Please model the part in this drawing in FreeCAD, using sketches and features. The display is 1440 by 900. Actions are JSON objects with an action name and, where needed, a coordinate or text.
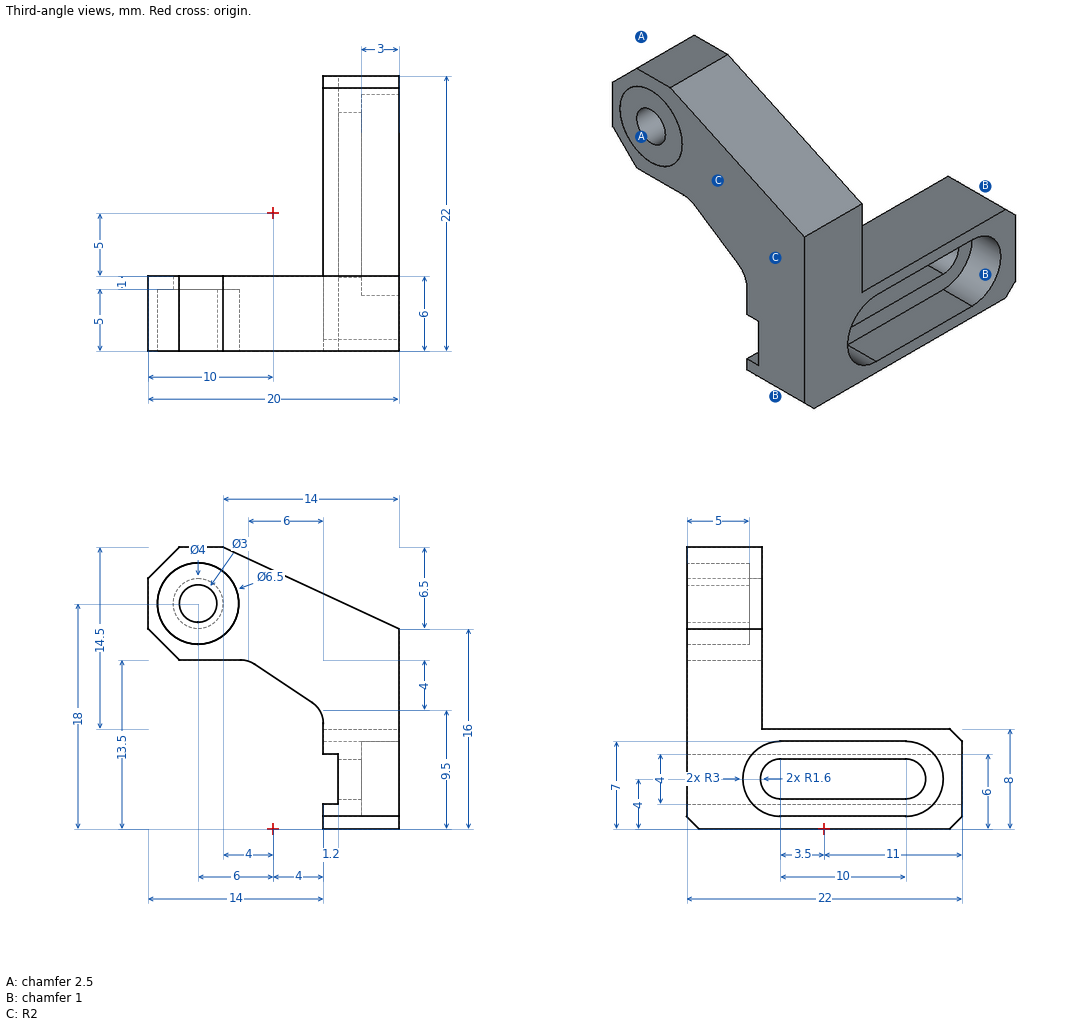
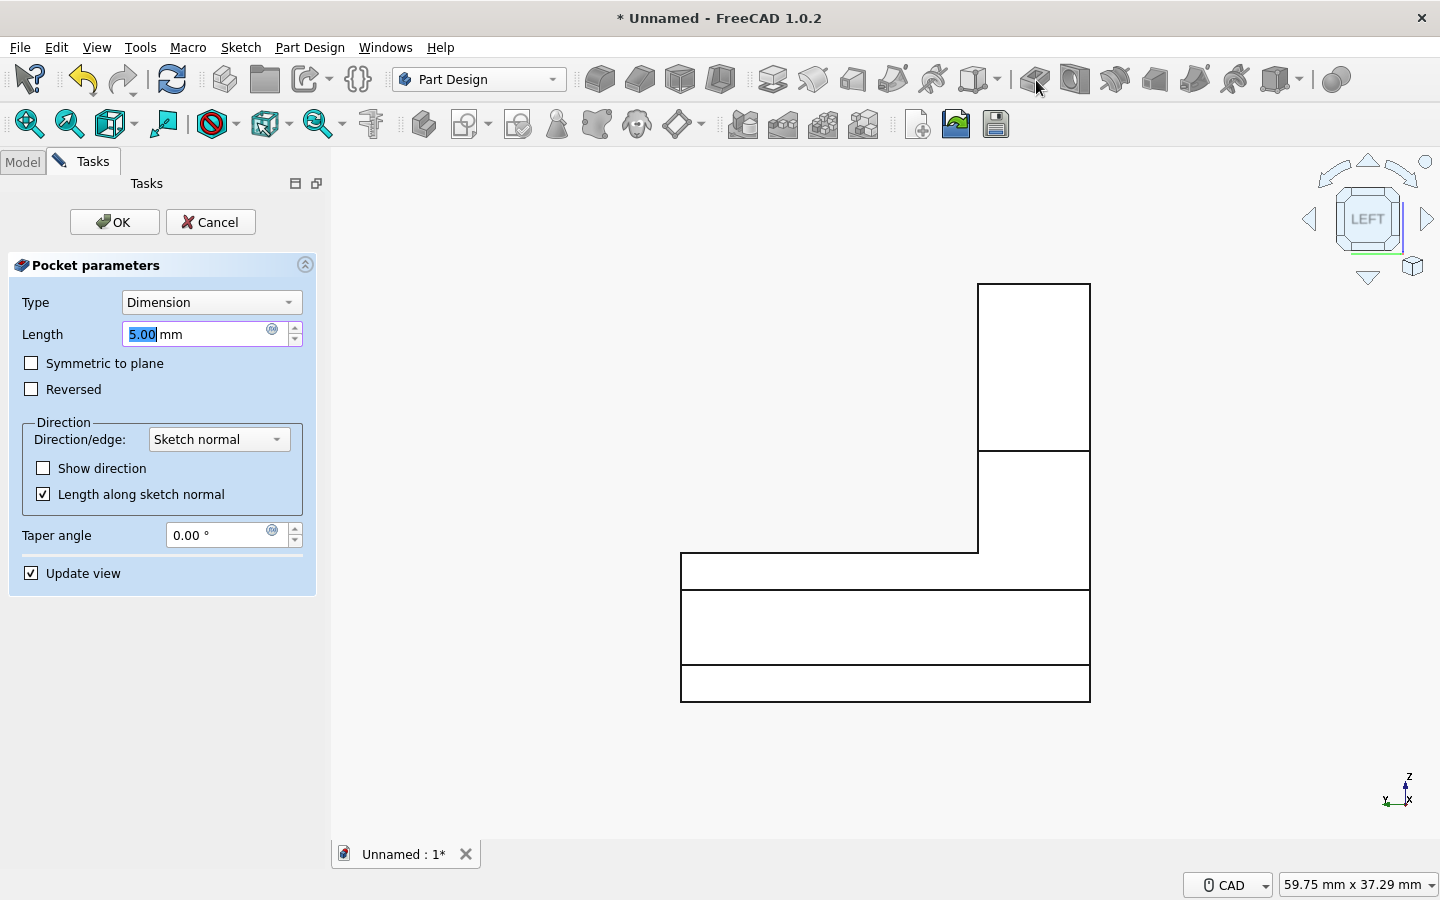
{"action": "type", "text": "1.2"}
{"action": "key", "text": "Tab"}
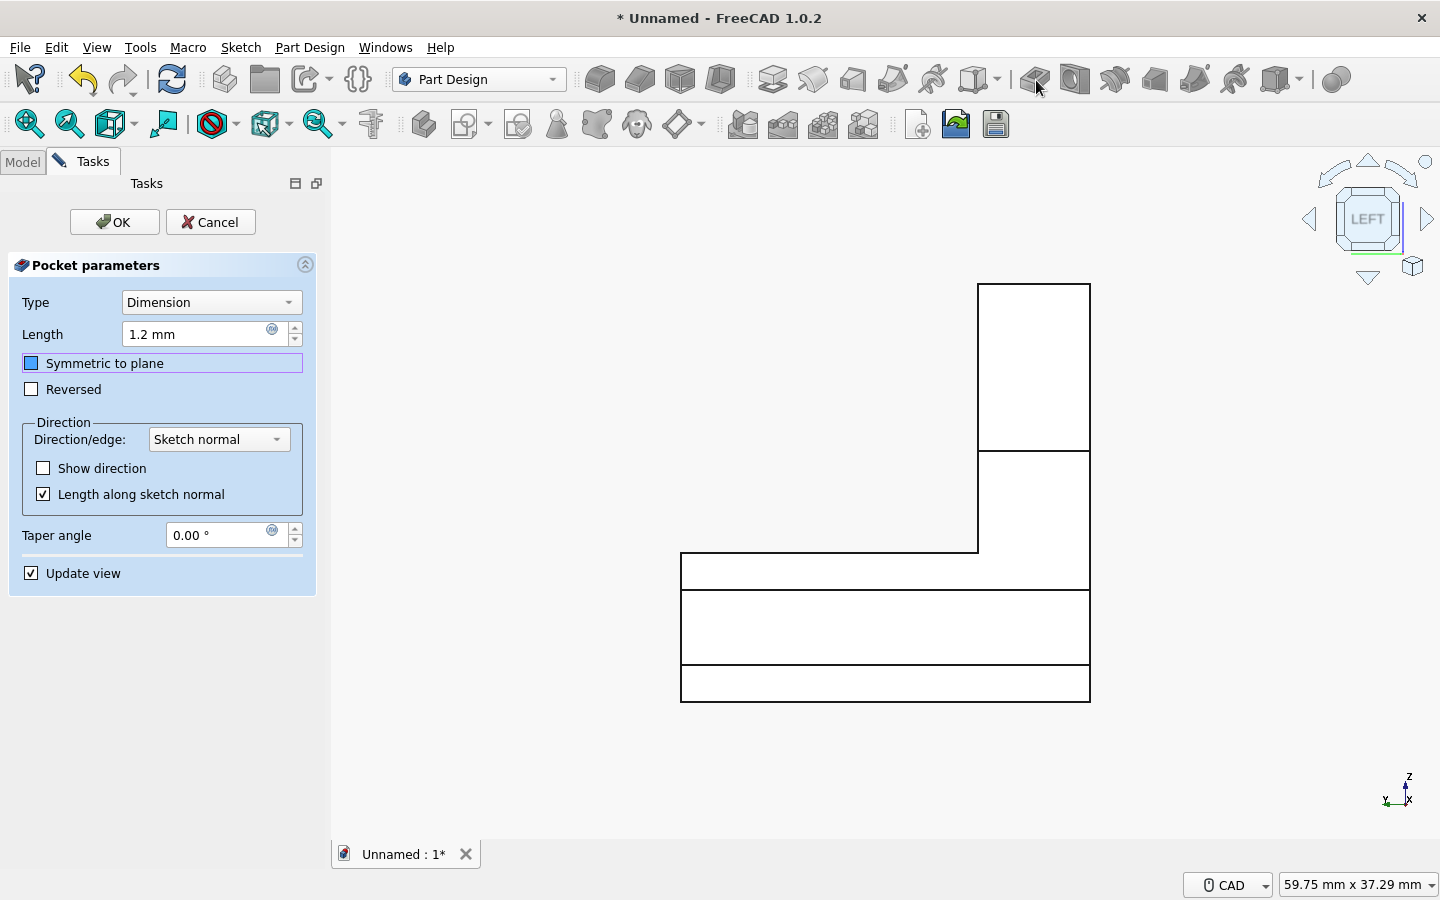
{"action": "left_click", "coordinate": [115, 222]}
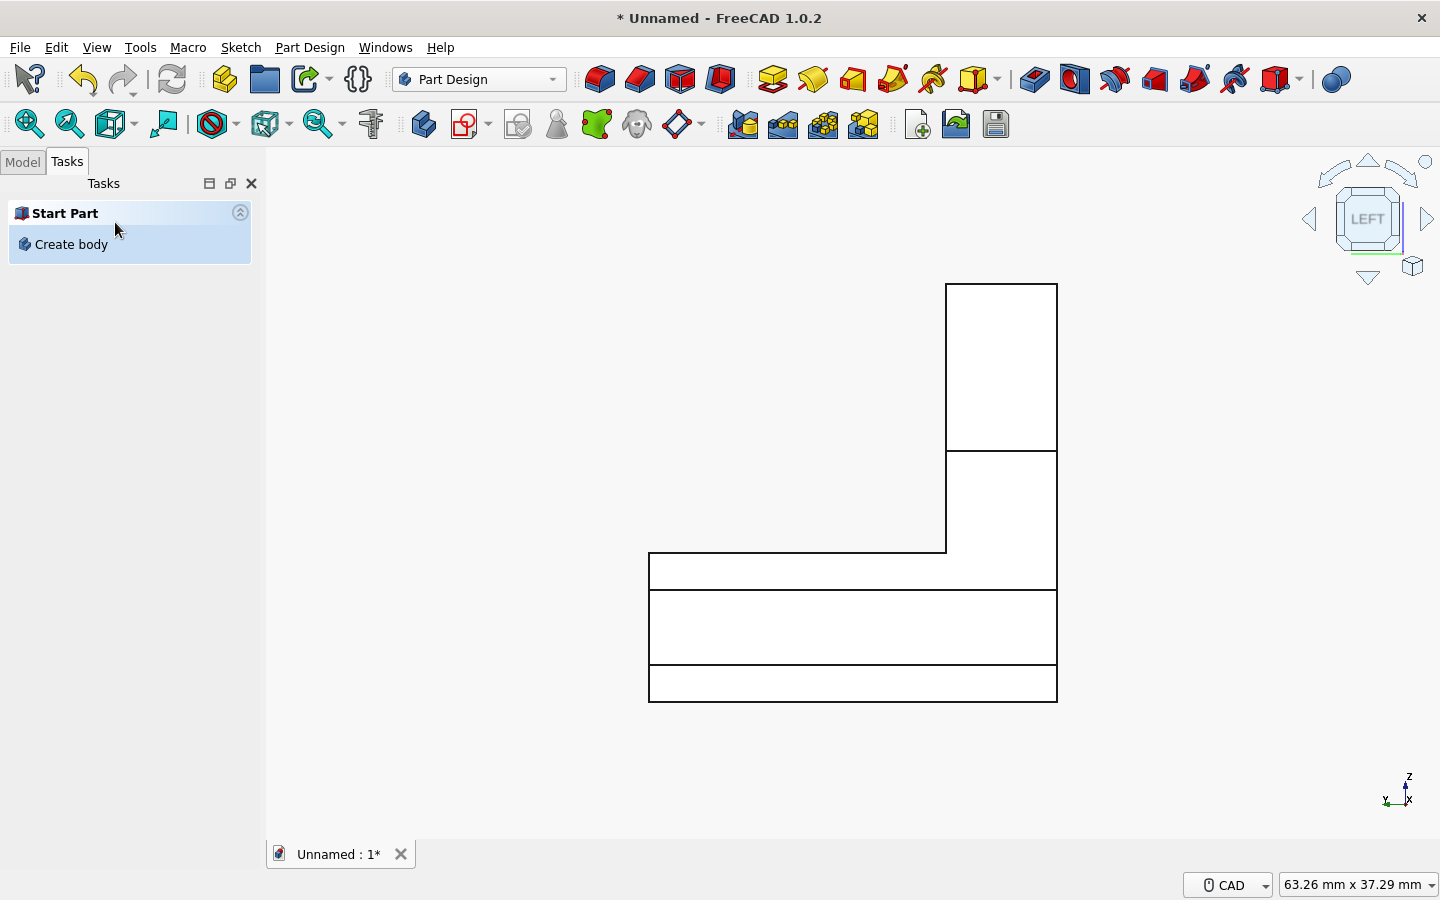
{"action": "key", "text": "0"}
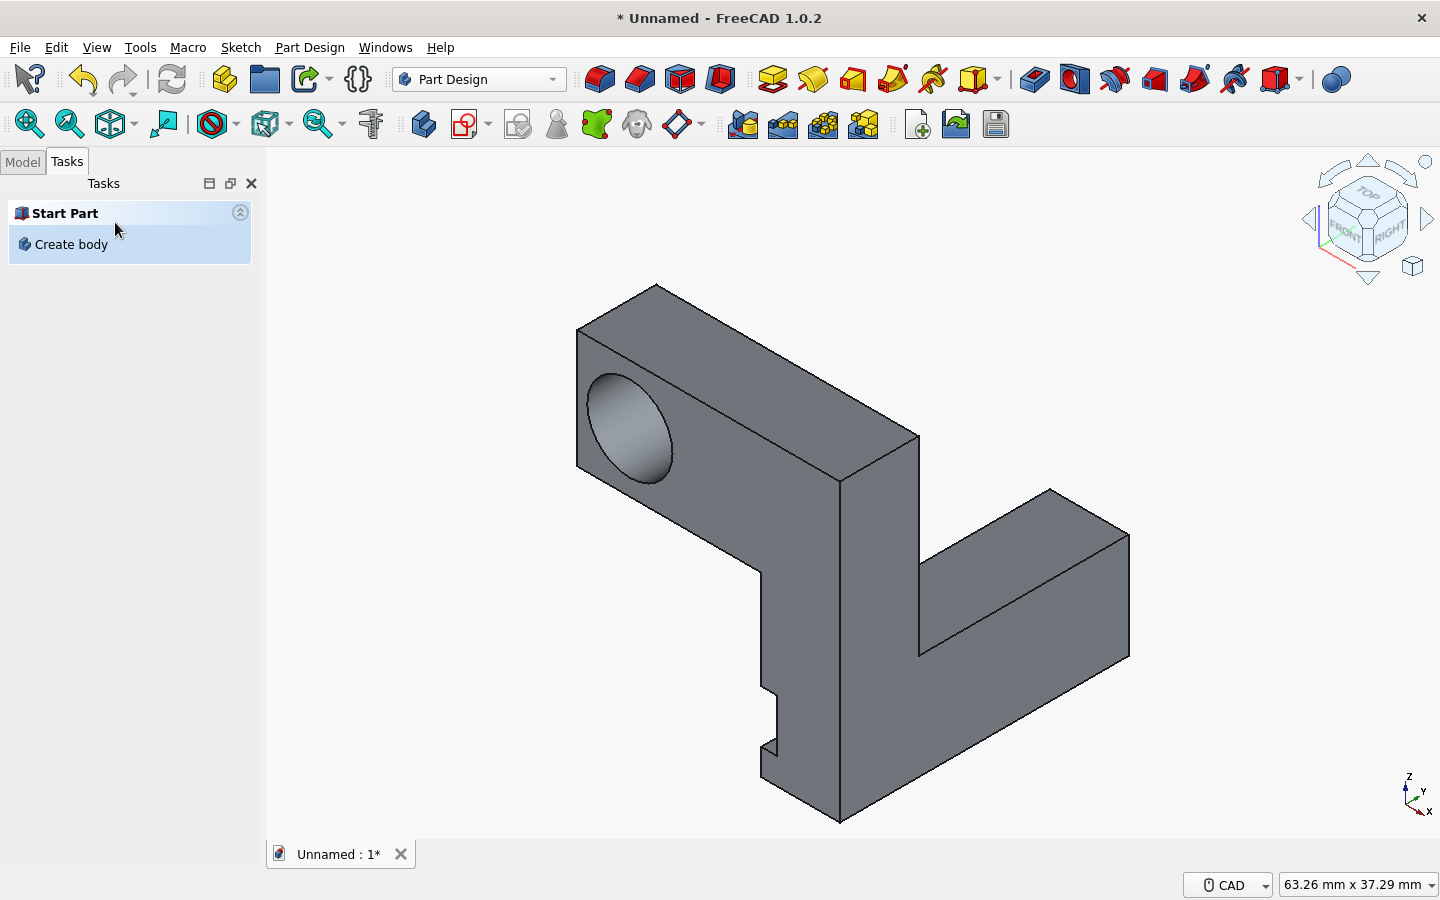
{"action": "left_click", "coordinate": [784, 521]}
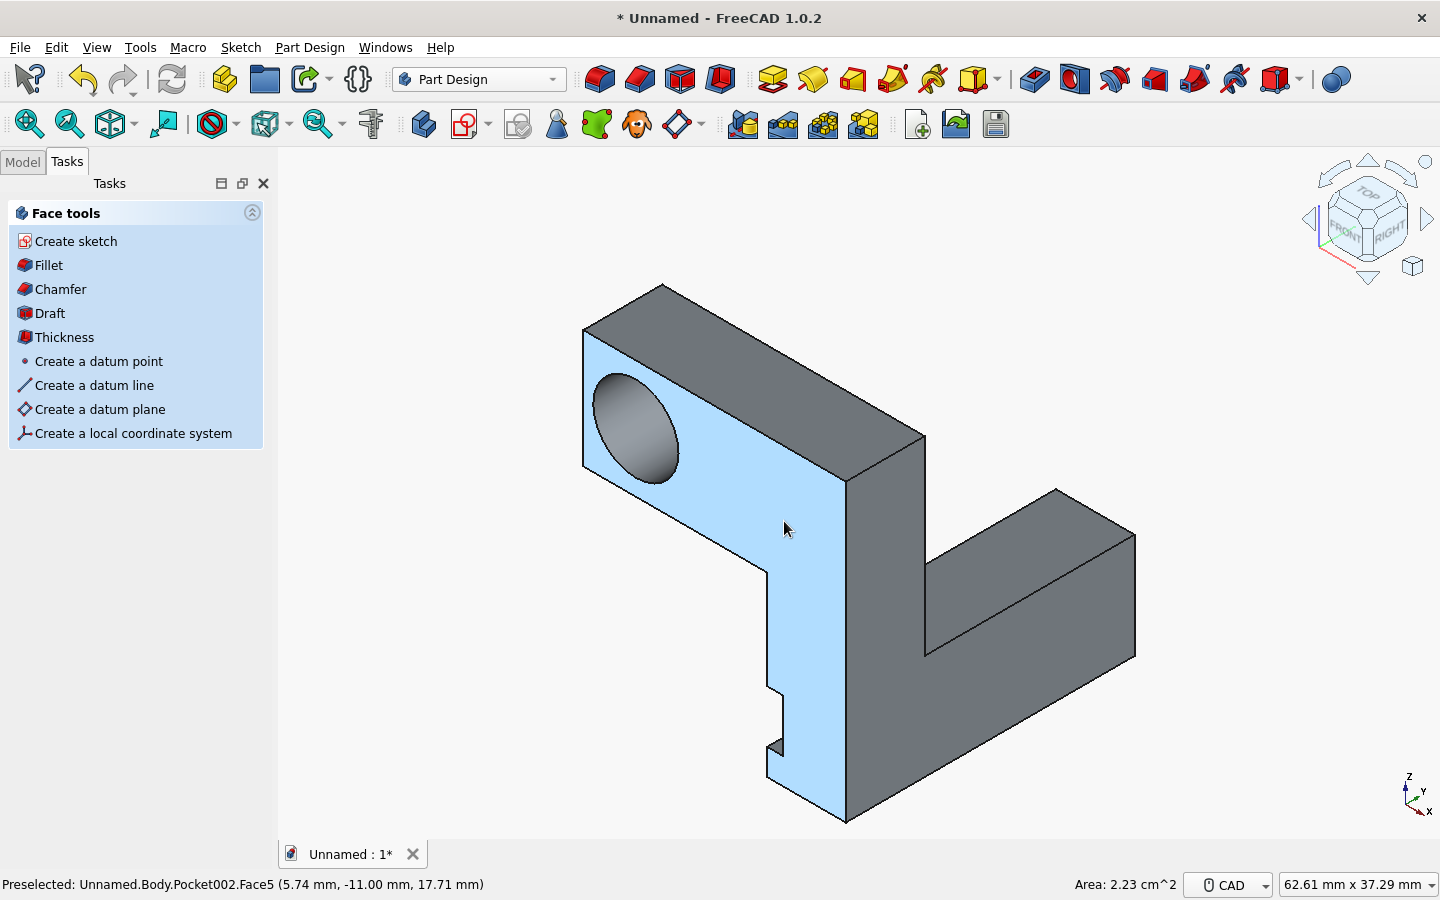
{"action": "left_click", "coordinate": [464, 124]}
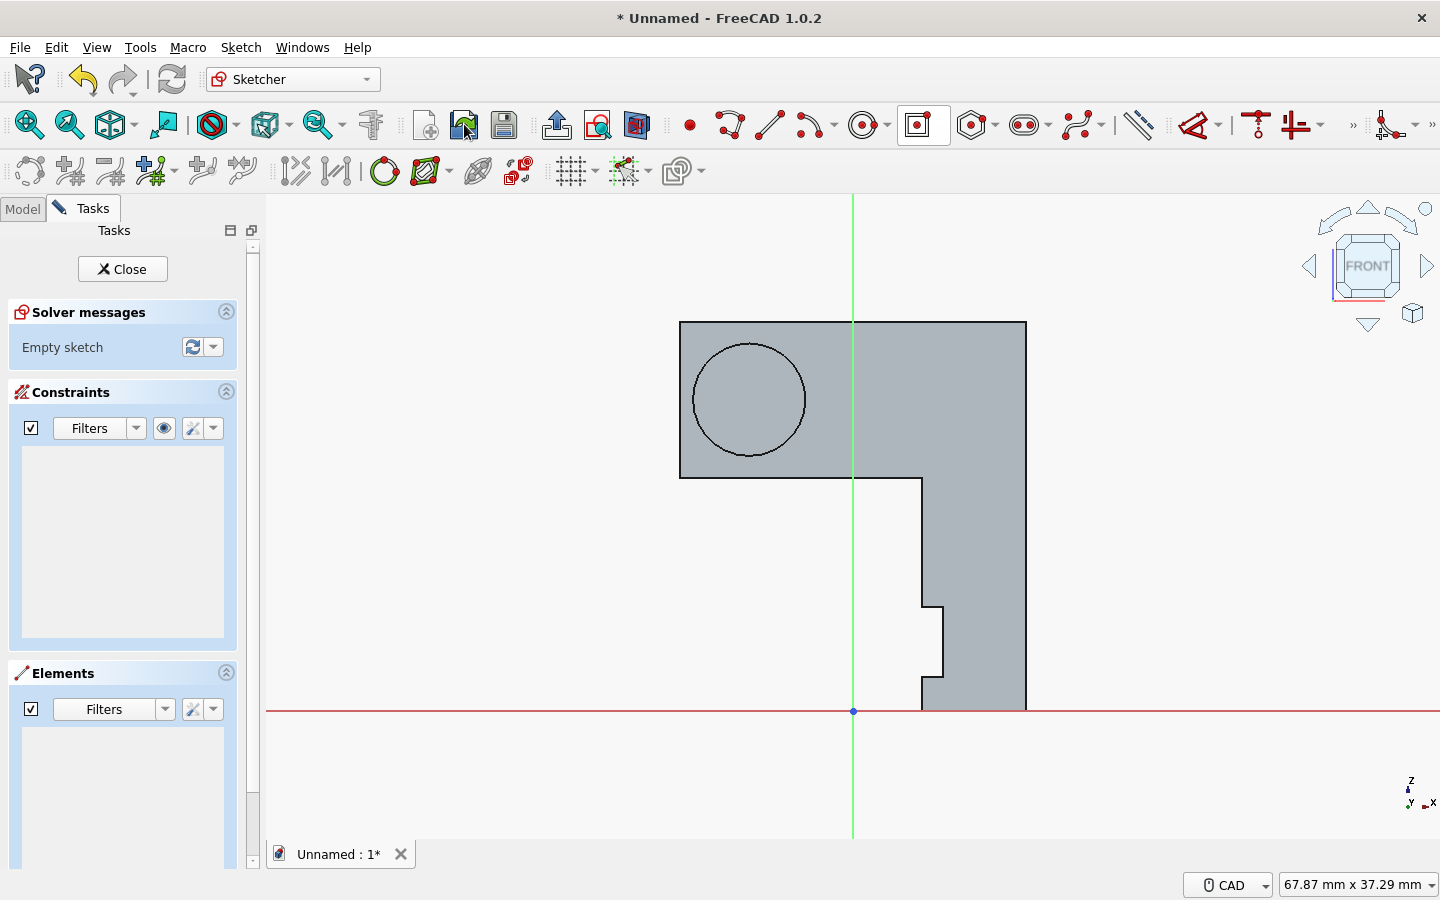
{"action": "left_click", "coordinate": [730, 126]}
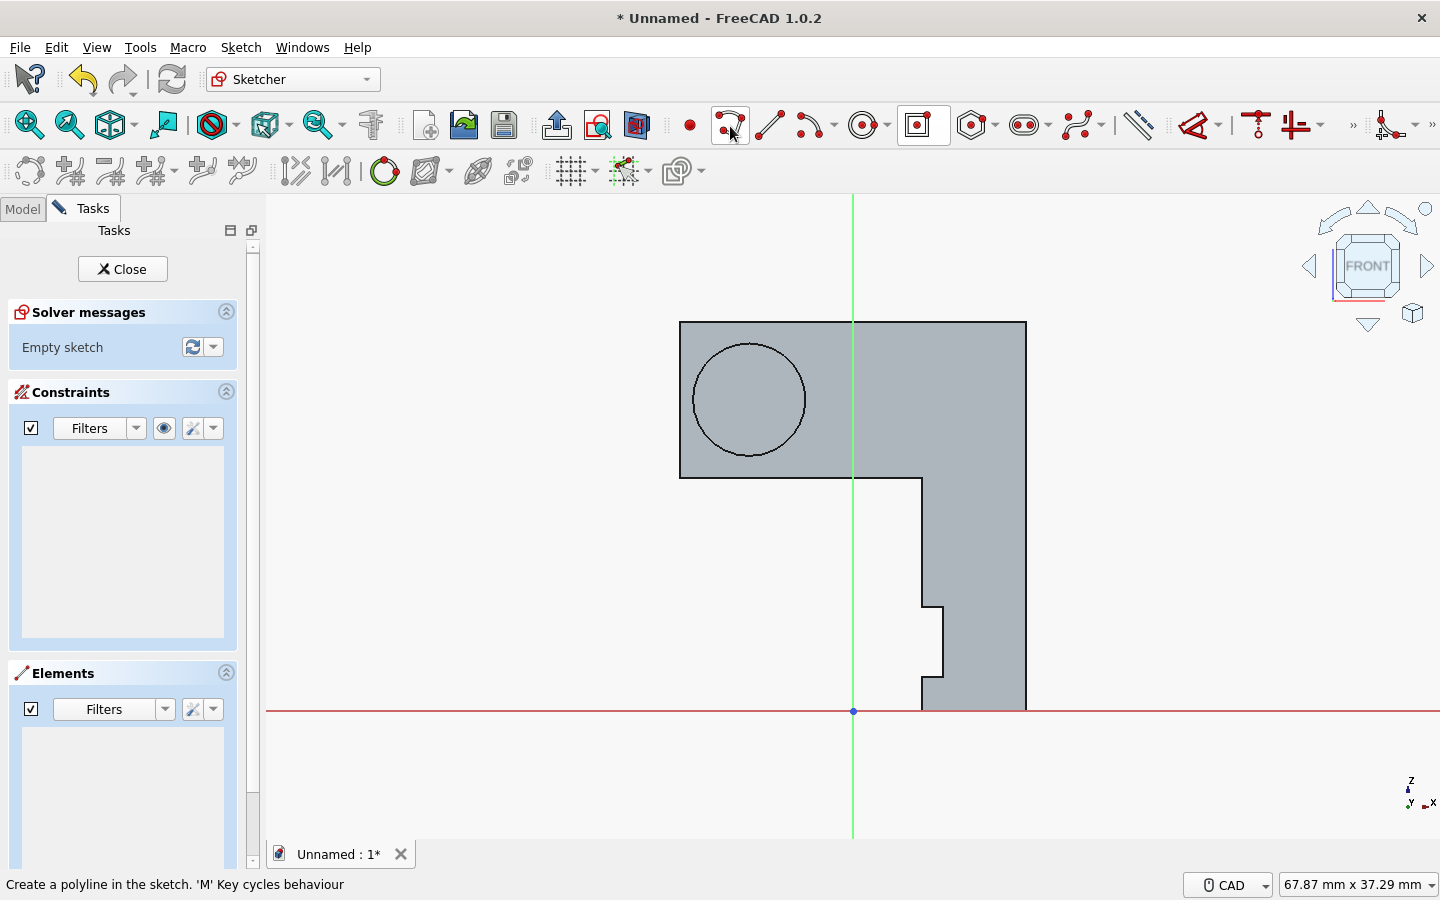
{"action": "left_click", "coordinate": [1026, 434]}
{"action": "left_click", "coordinate": [1026, 322]}
{"action": "left_click", "coordinate": [784, 322]}
{"action": "left_click", "coordinate": [1026, 435]}
{"action": "key", "text": "Escape"}
{"action": "key", "text": "Escape"}